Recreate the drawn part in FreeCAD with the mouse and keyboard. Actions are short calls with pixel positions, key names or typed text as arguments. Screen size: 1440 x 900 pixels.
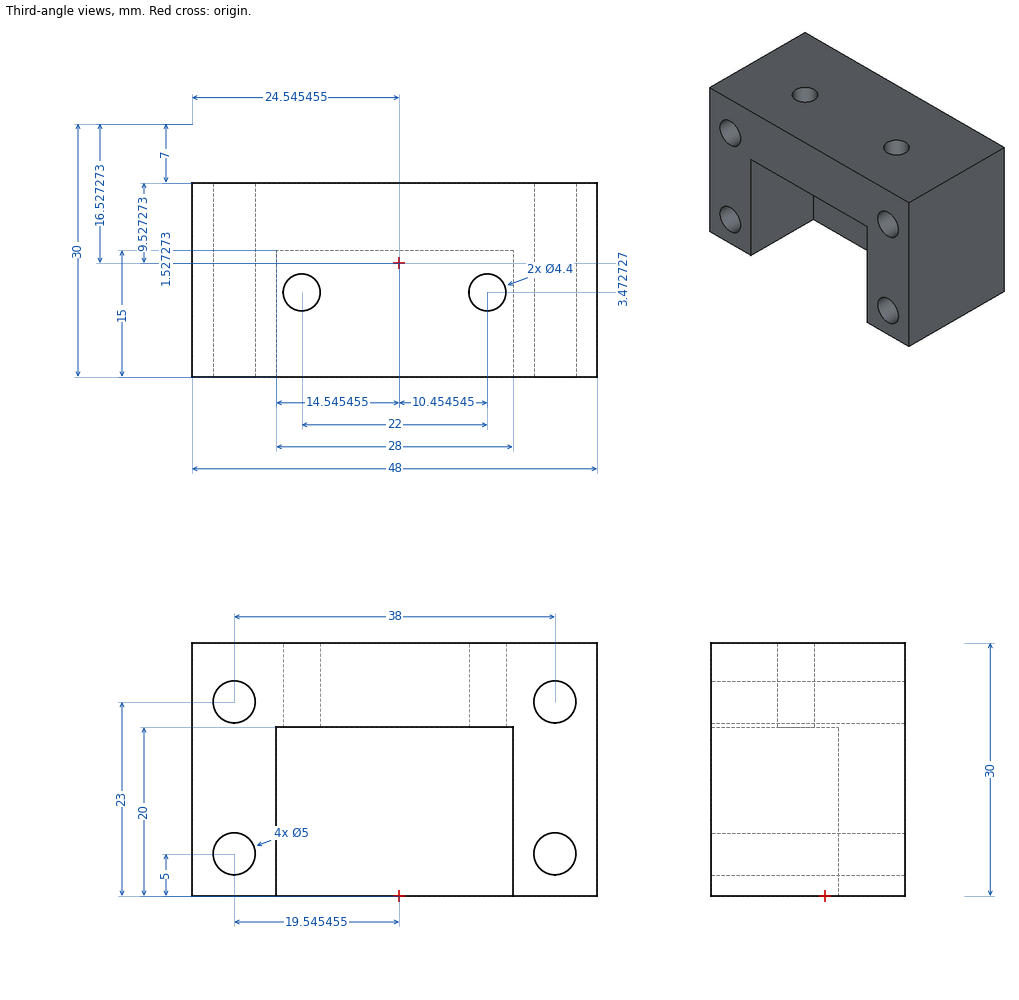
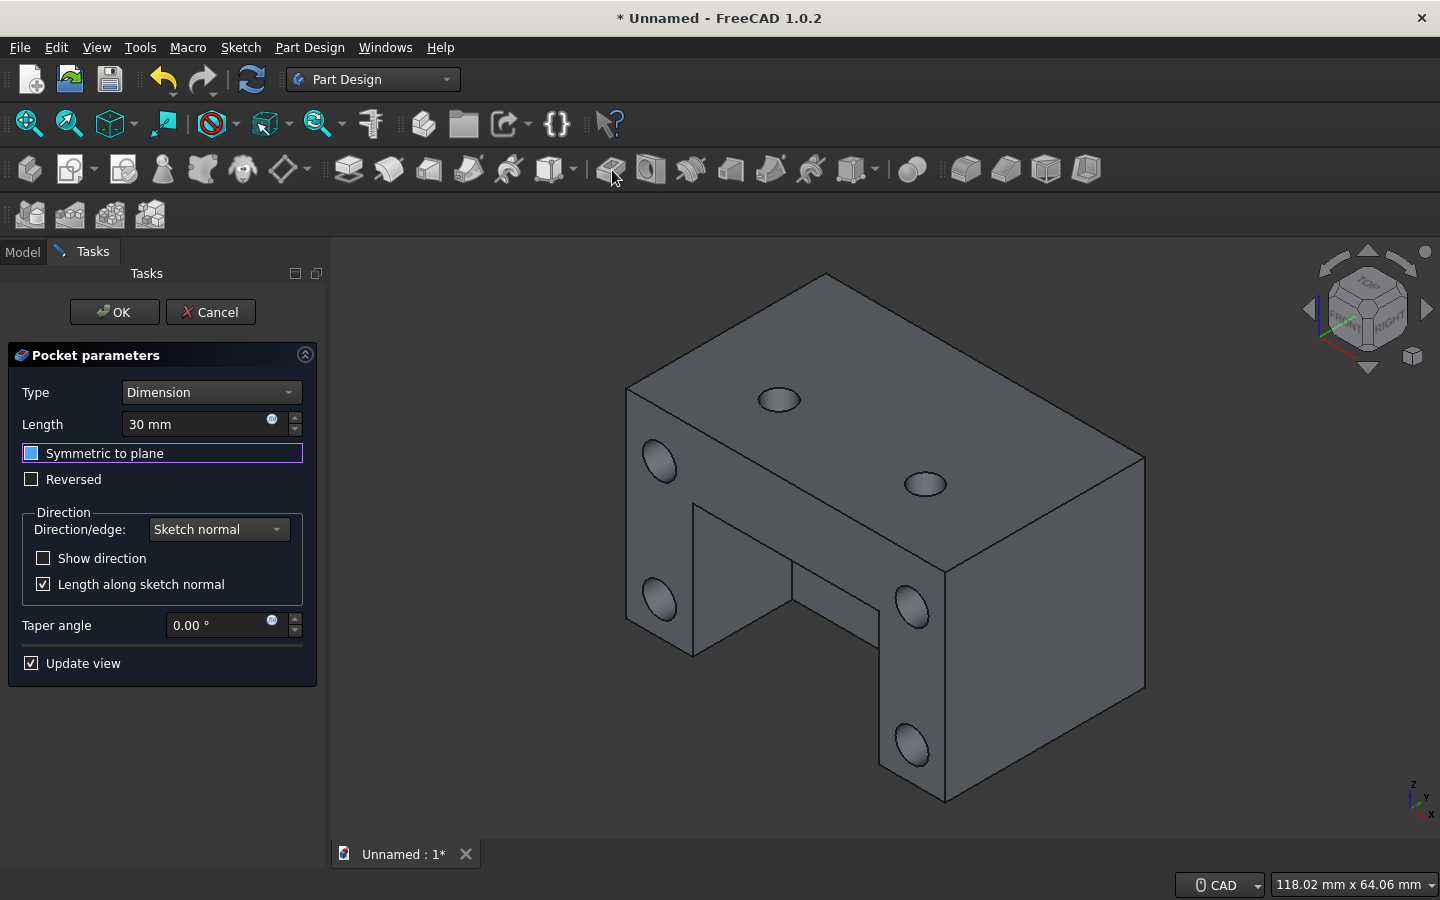
click(115, 312)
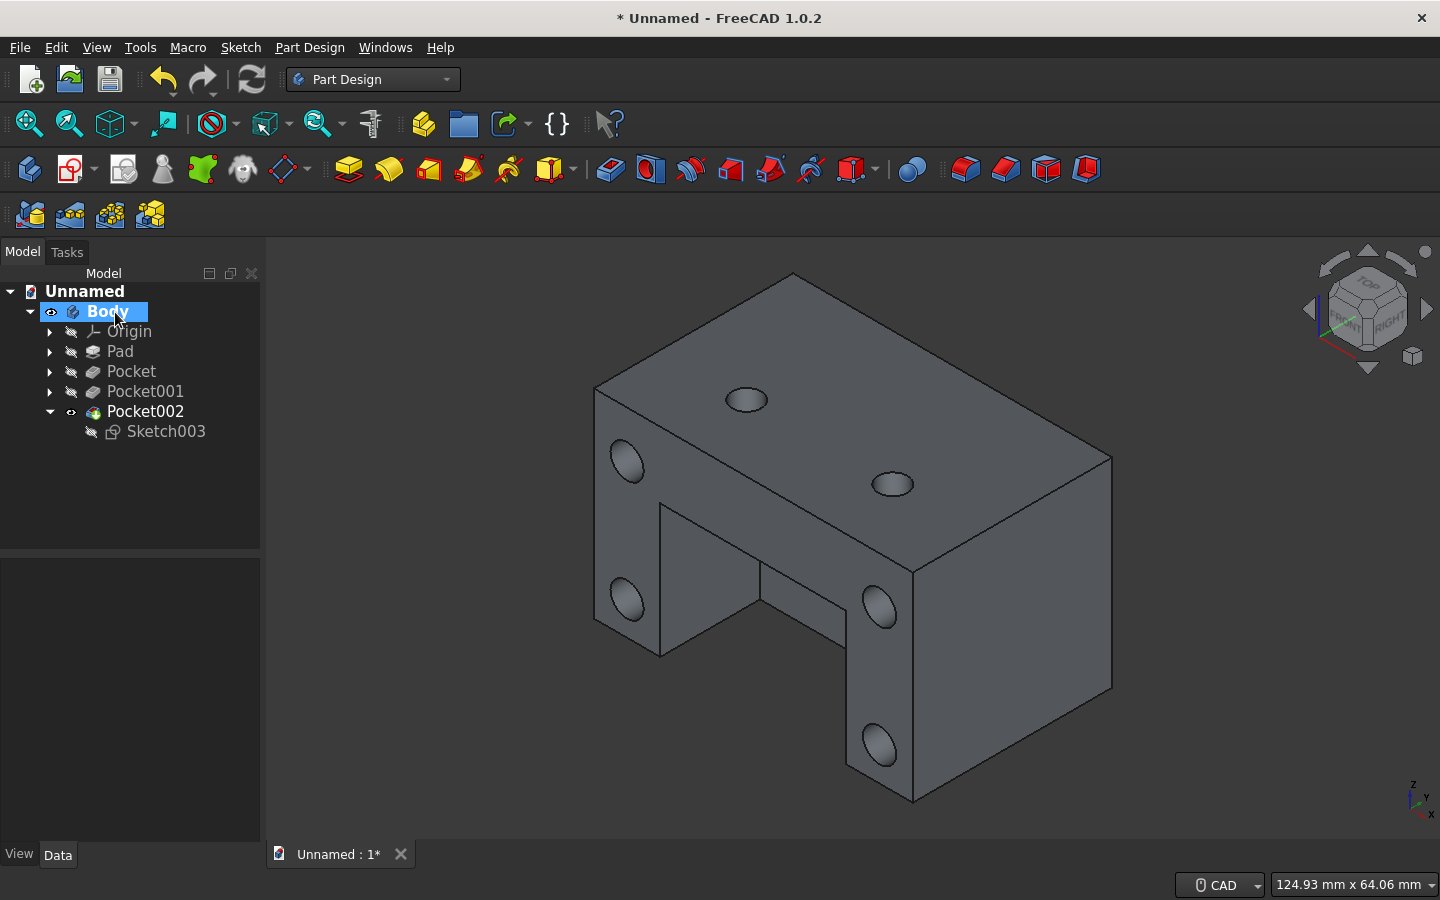
key(5)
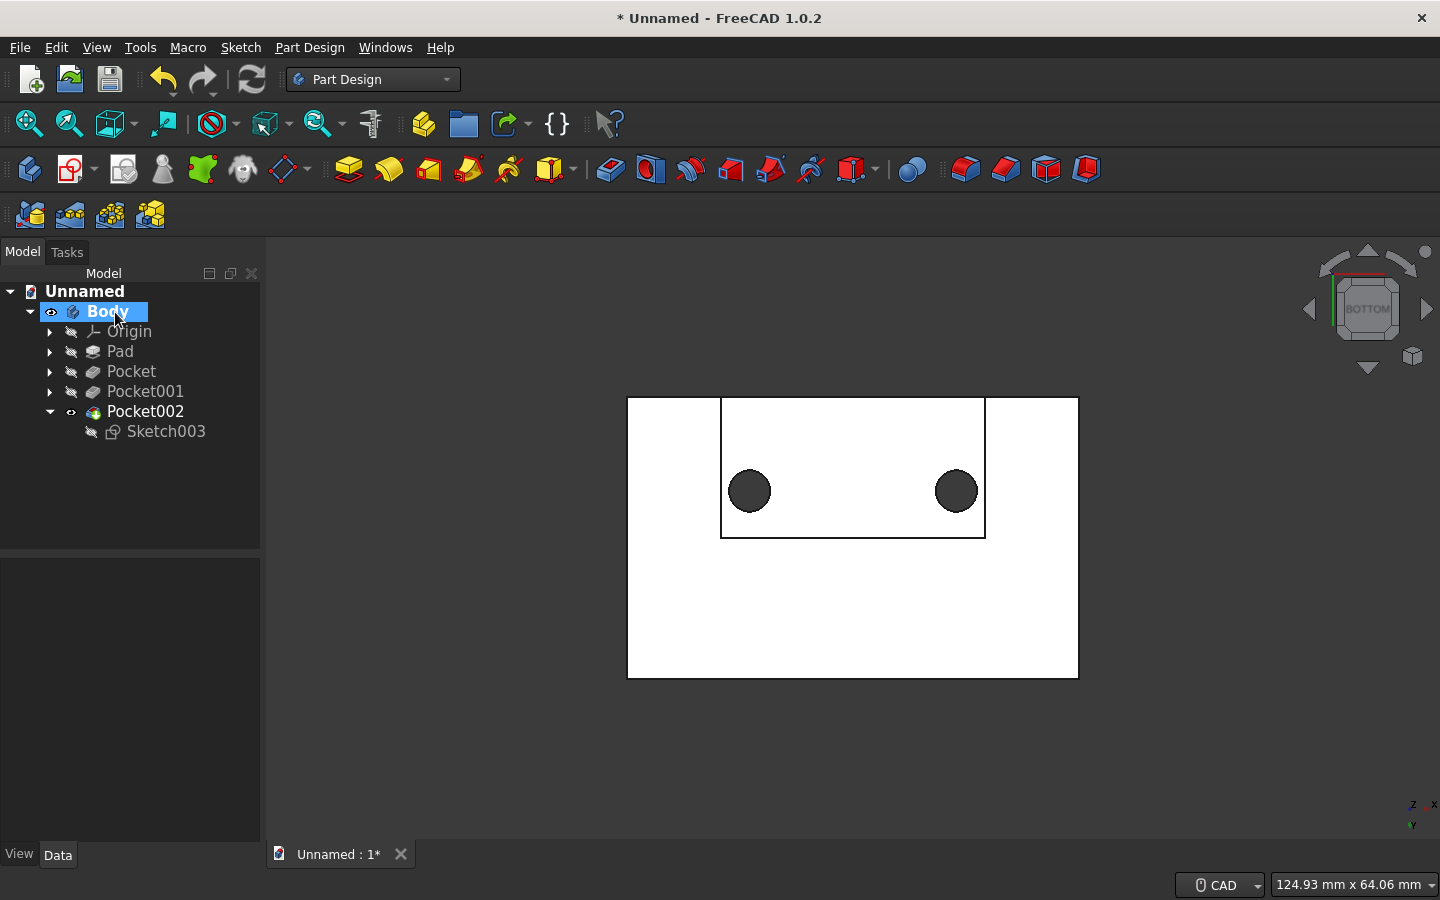
click(982, 618)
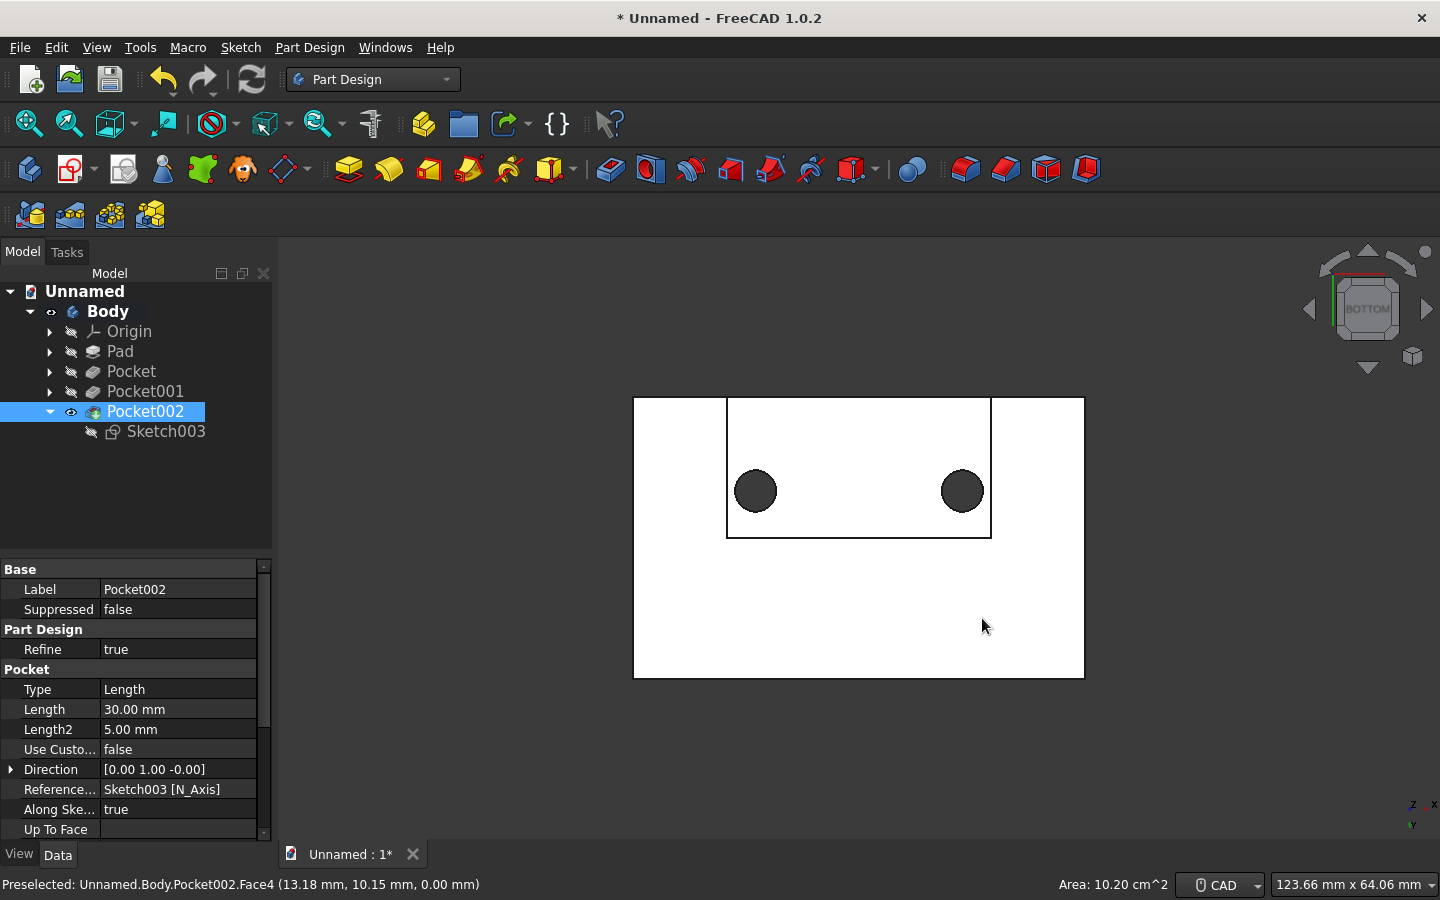
click(70, 170)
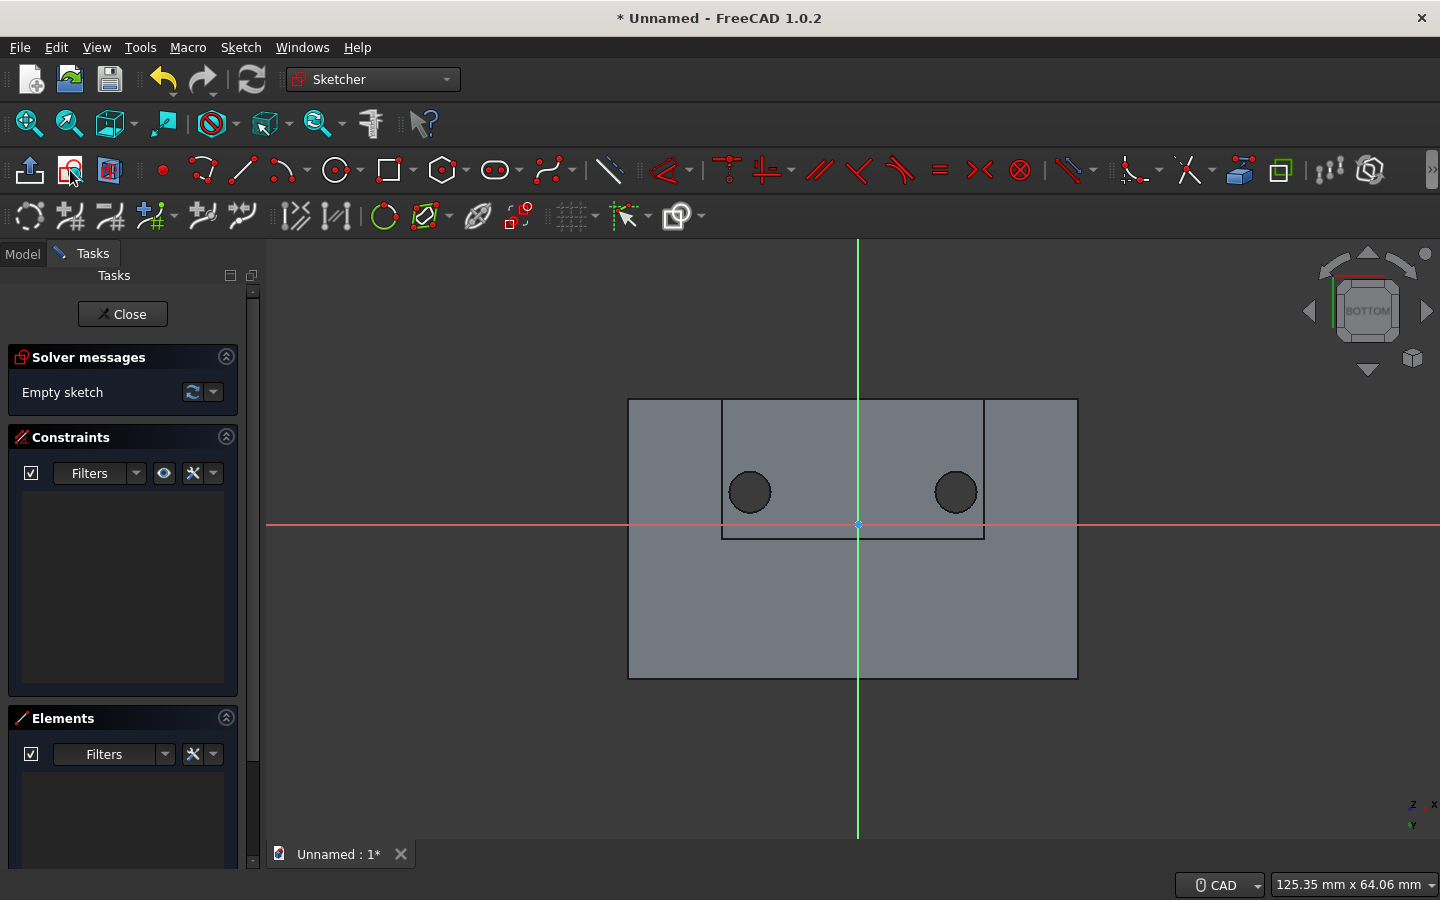
scroll(992, 730, up, 2)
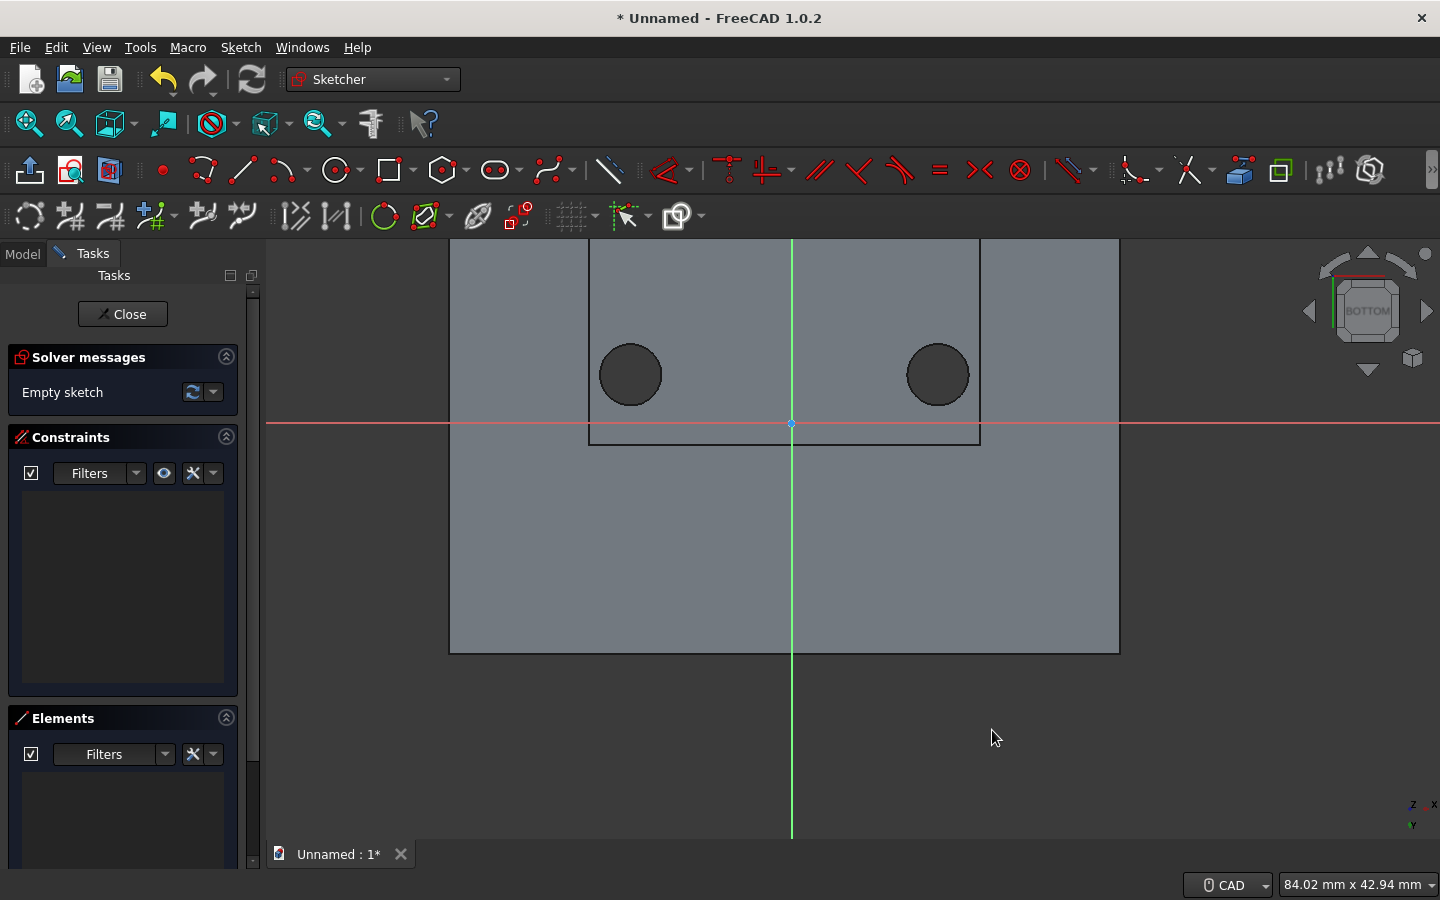
click(390, 170)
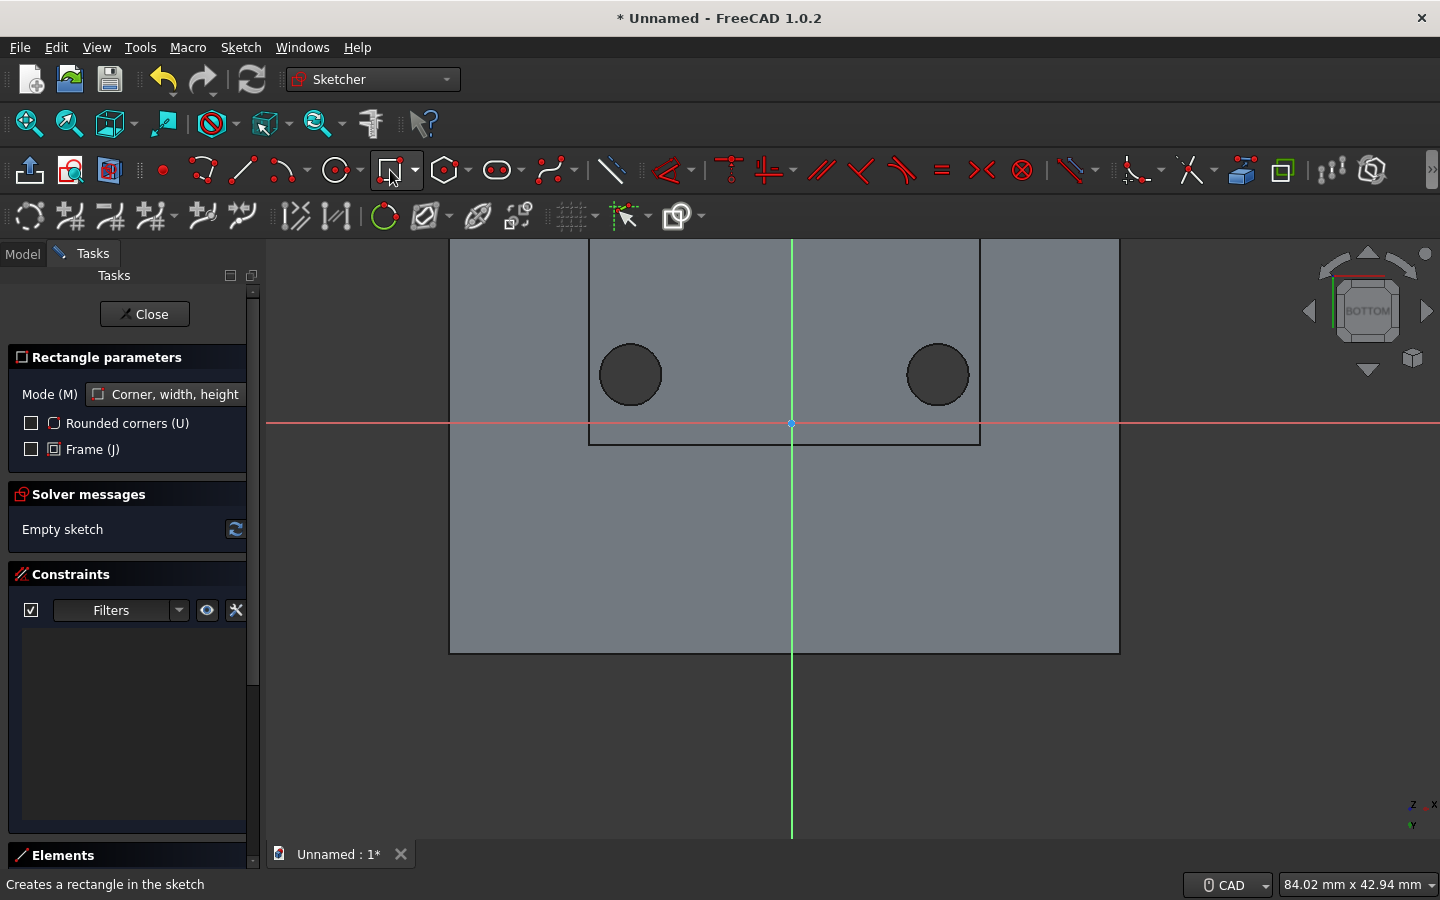
click(449, 556)
click(1120, 654)
key(Escape)